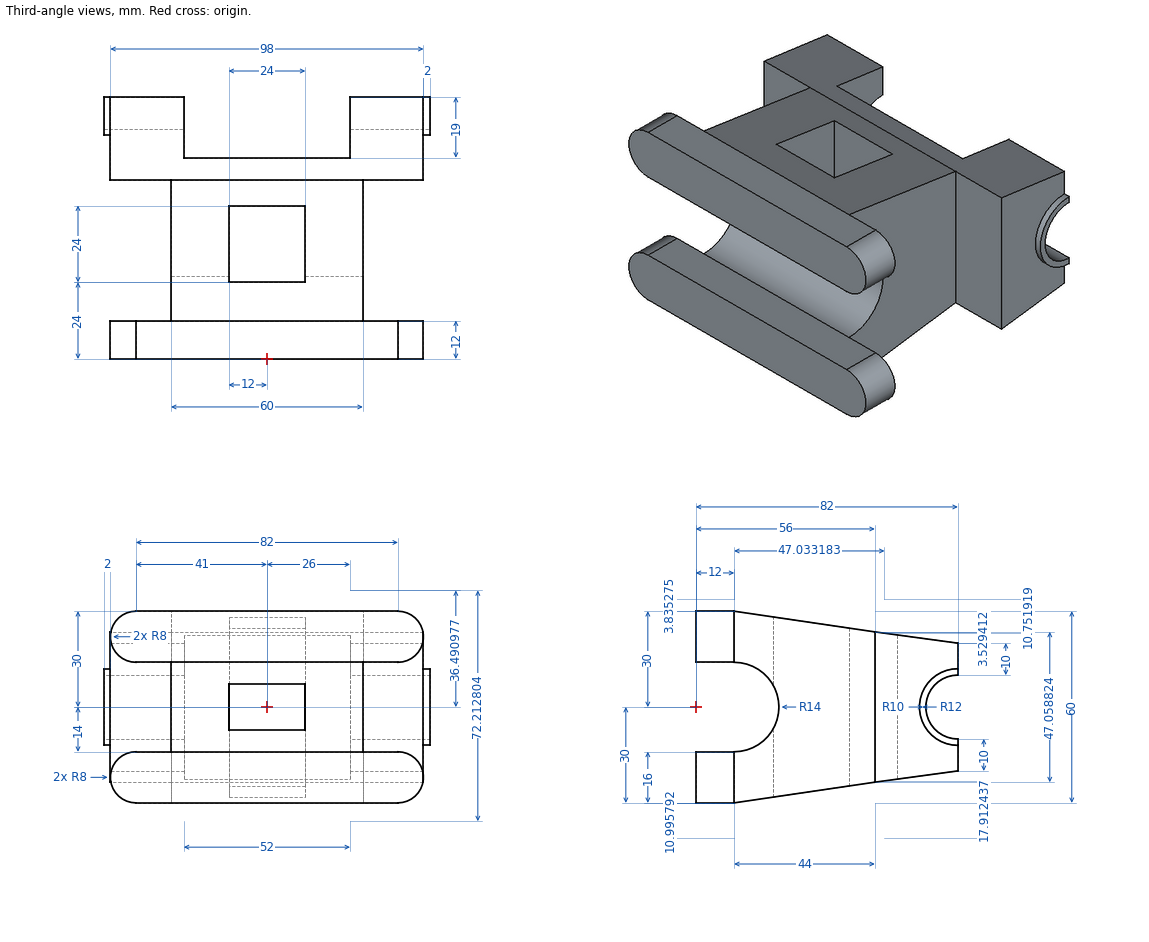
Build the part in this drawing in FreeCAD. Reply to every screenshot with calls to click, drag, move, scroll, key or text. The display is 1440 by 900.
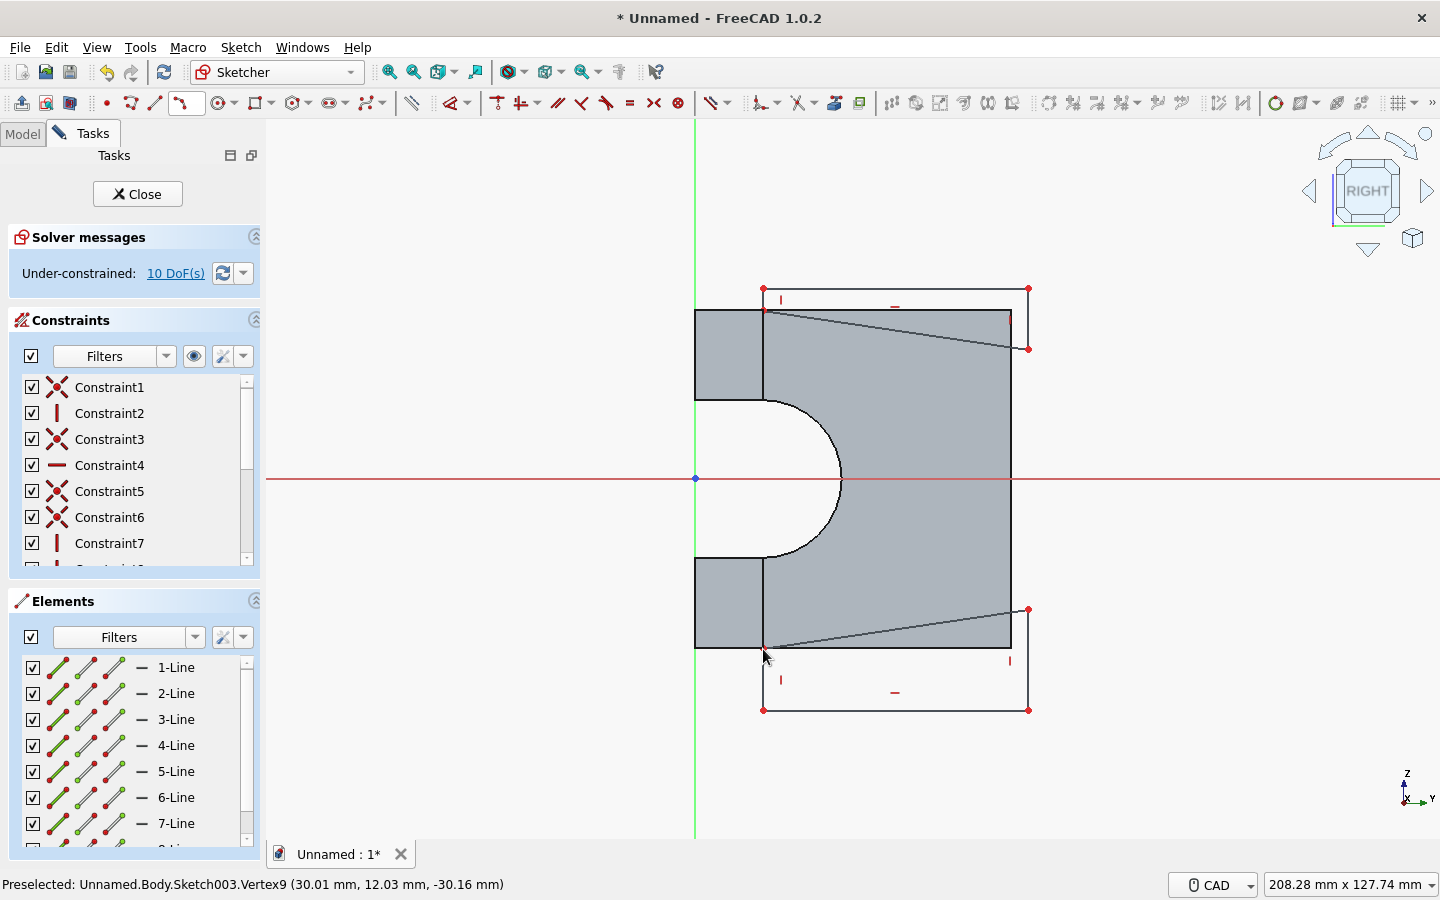
click(450, 104)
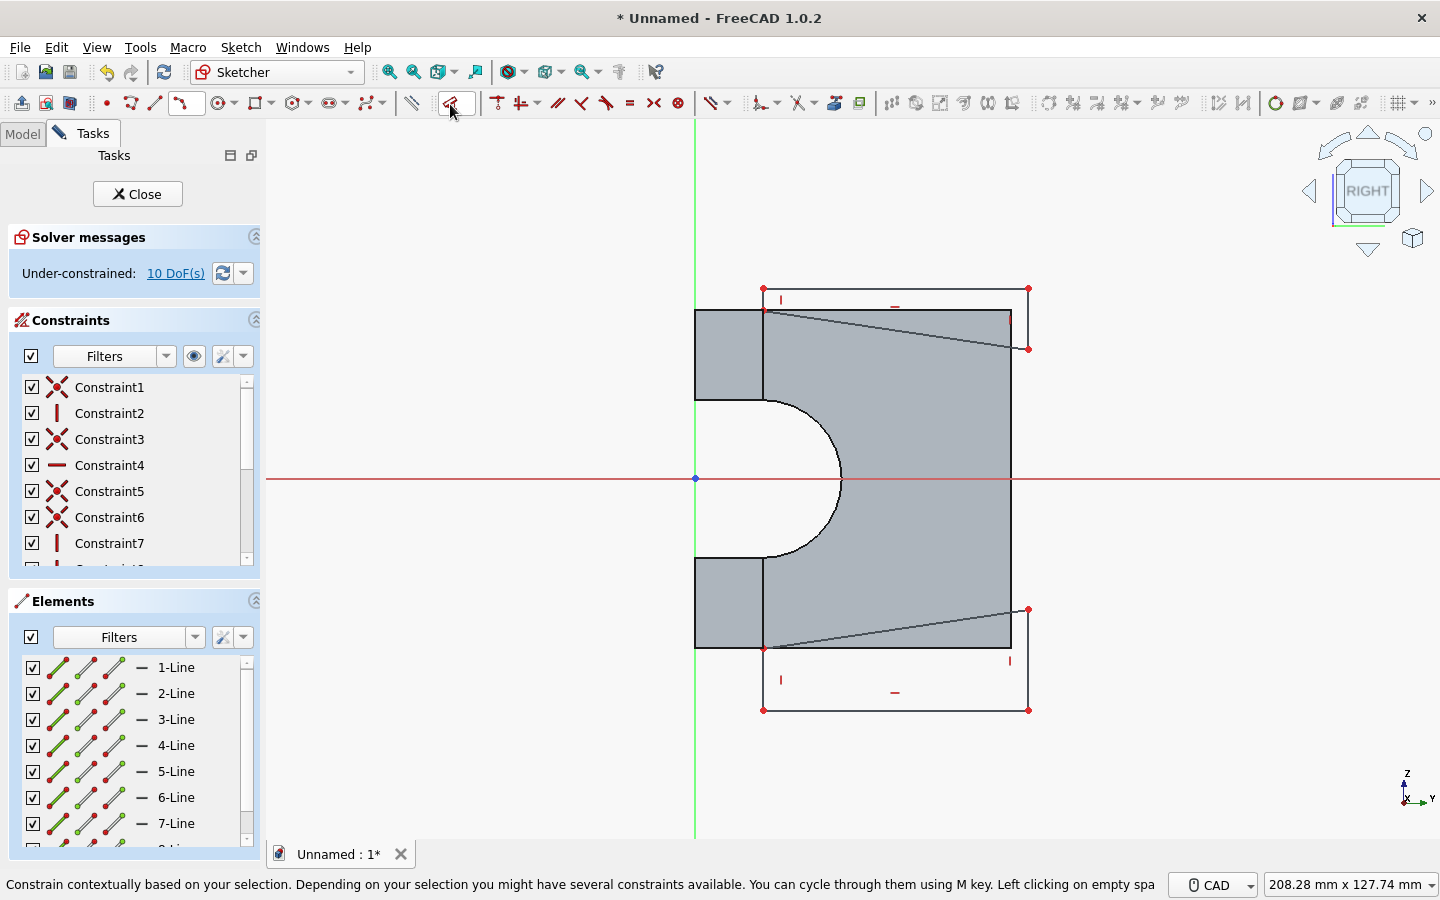
click(763, 311)
click(729, 277)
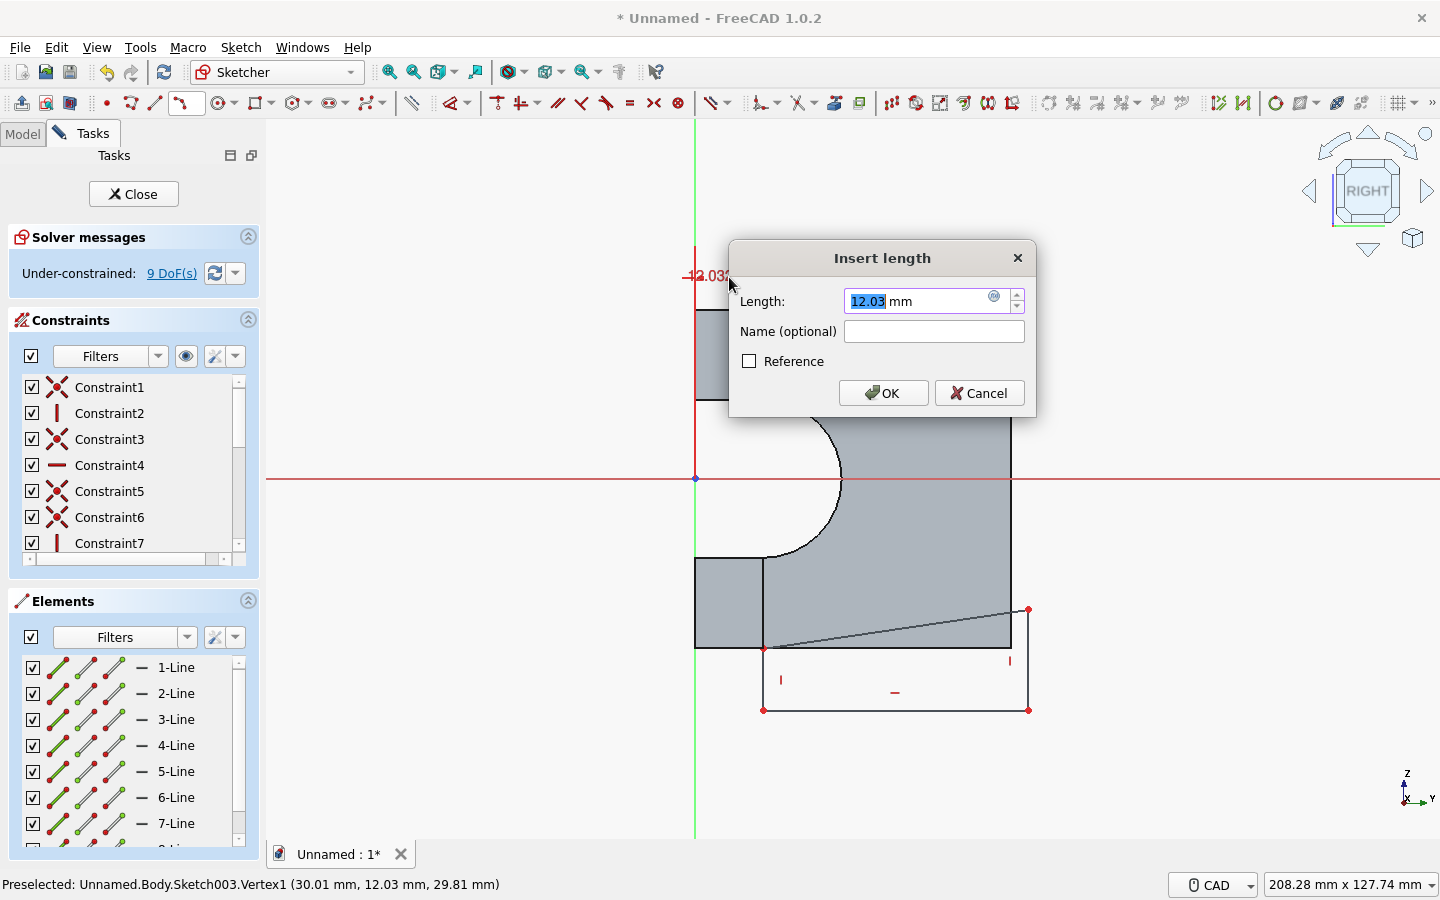
text(12)
key(Return)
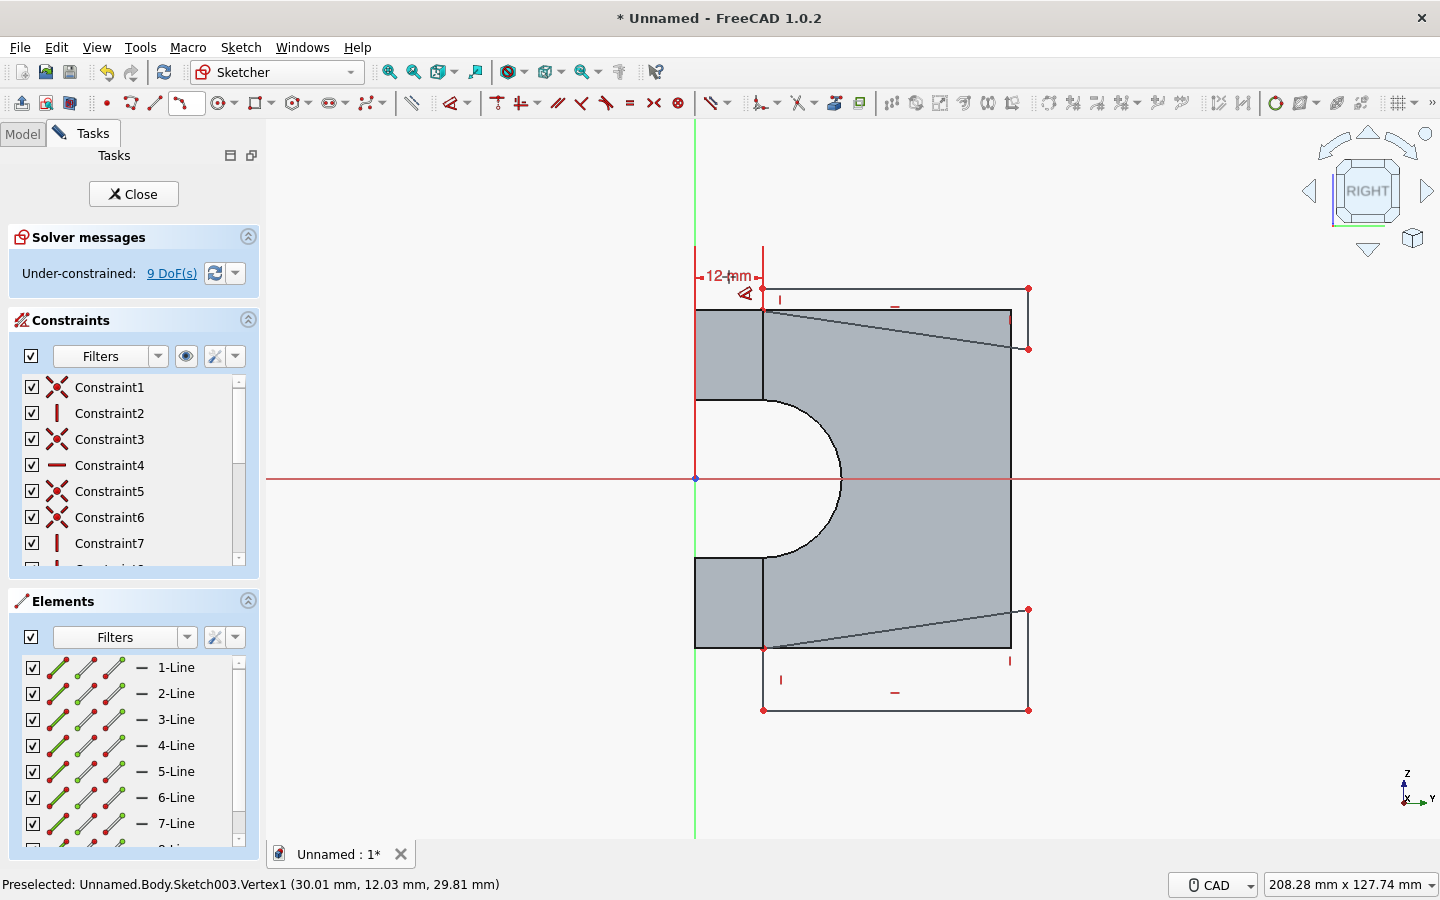
click(763, 311)
click(661, 395)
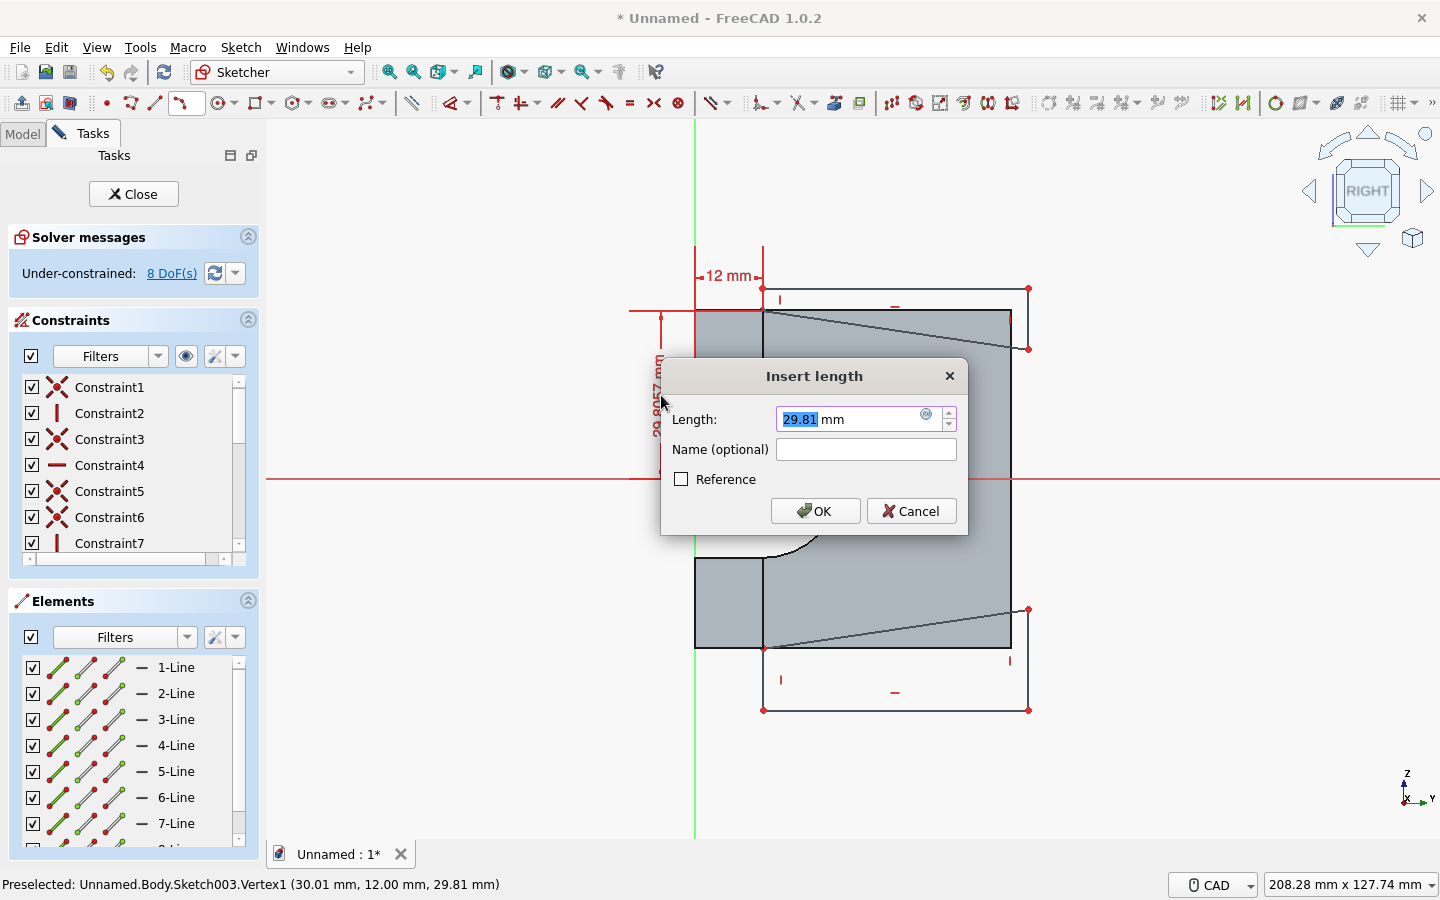
text(30)
key(Return)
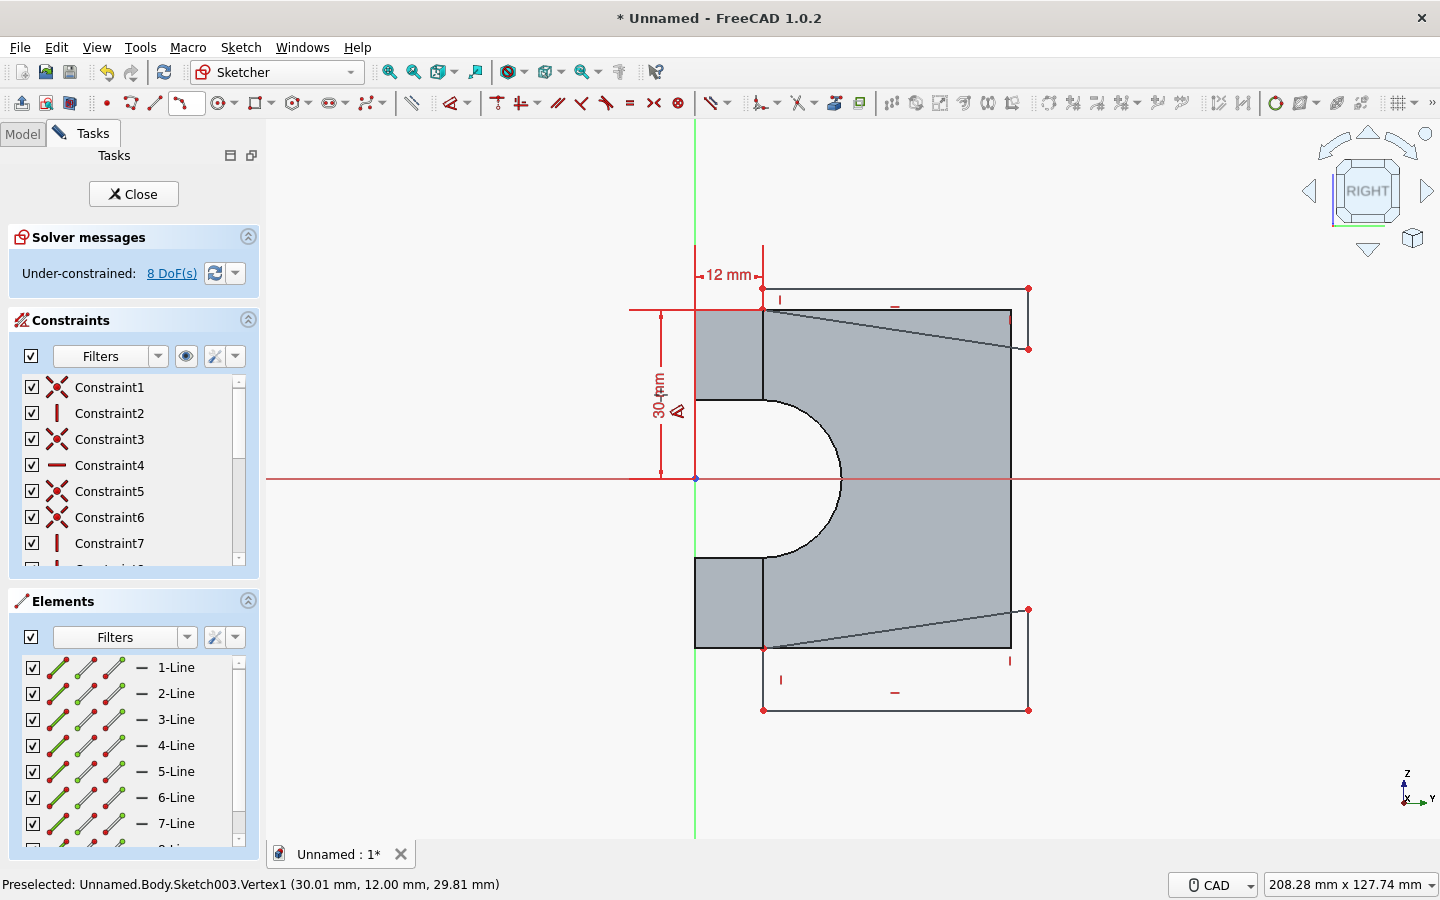
click(763, 649)
click(729, 683)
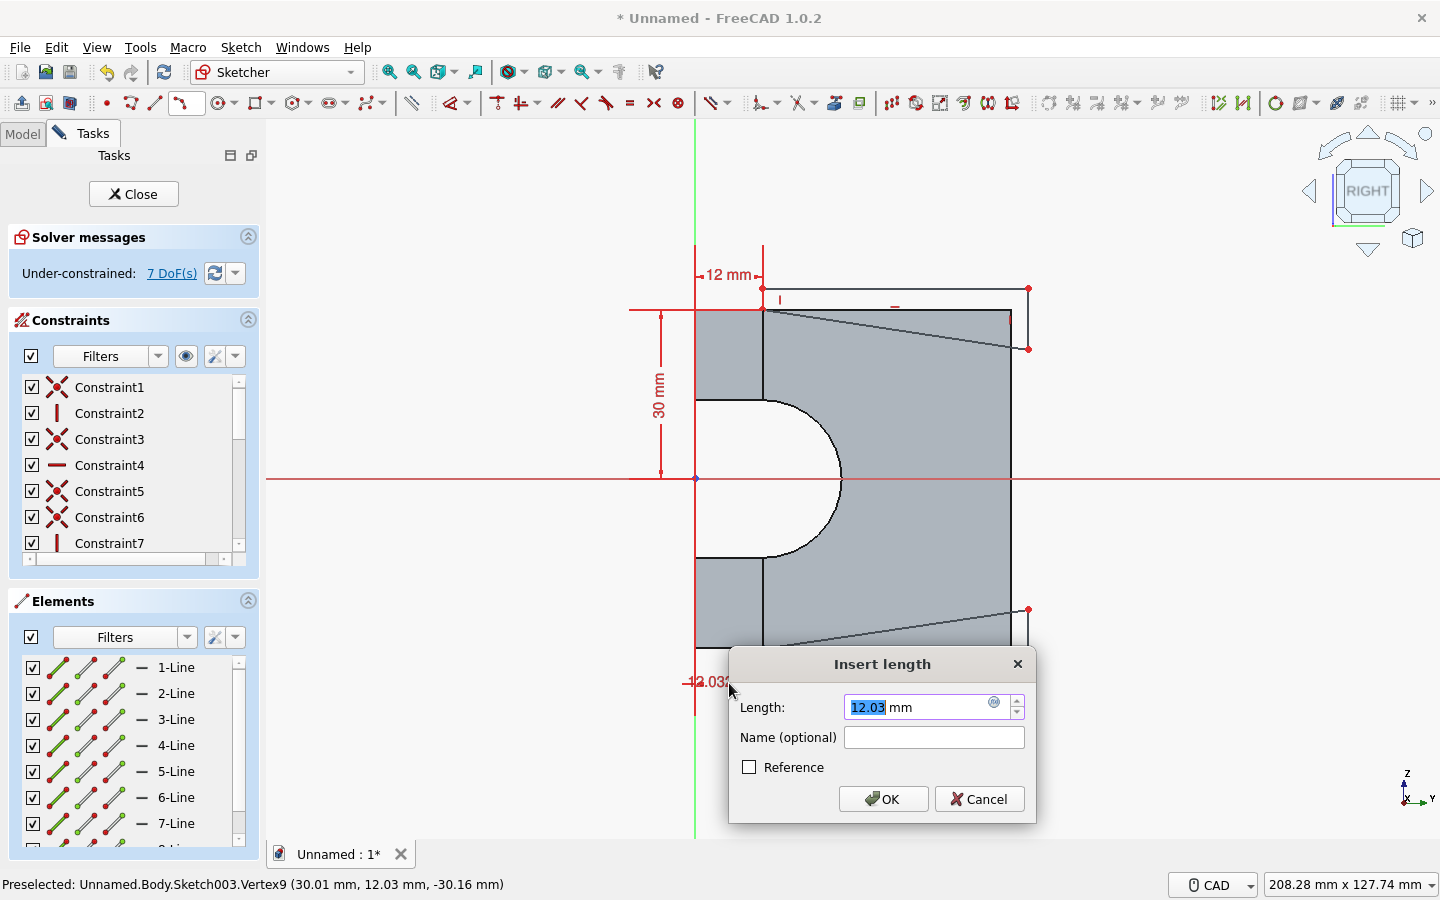
text(12)
key(Return)